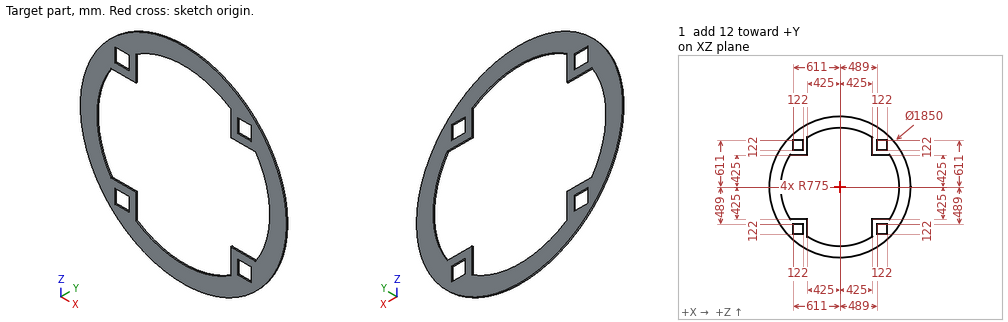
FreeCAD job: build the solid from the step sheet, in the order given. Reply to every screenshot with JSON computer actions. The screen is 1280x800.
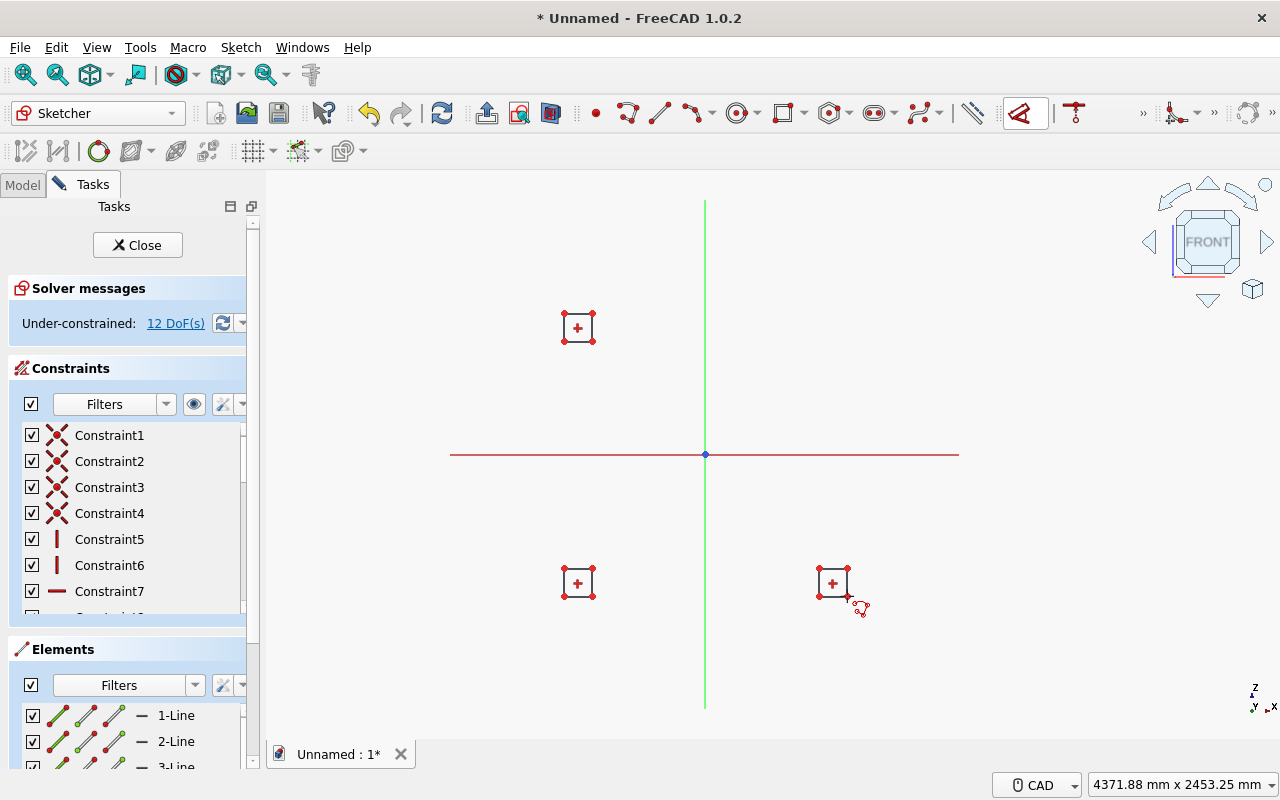
{"action": "left_click", "coordinate": [555, 553]}
{"action": "left_click", "coordinate": [607, 553]}
{"action": "left_click", "coordinate": [607, 605]}
{"action": "right_click", "coordinate": [607, 605]}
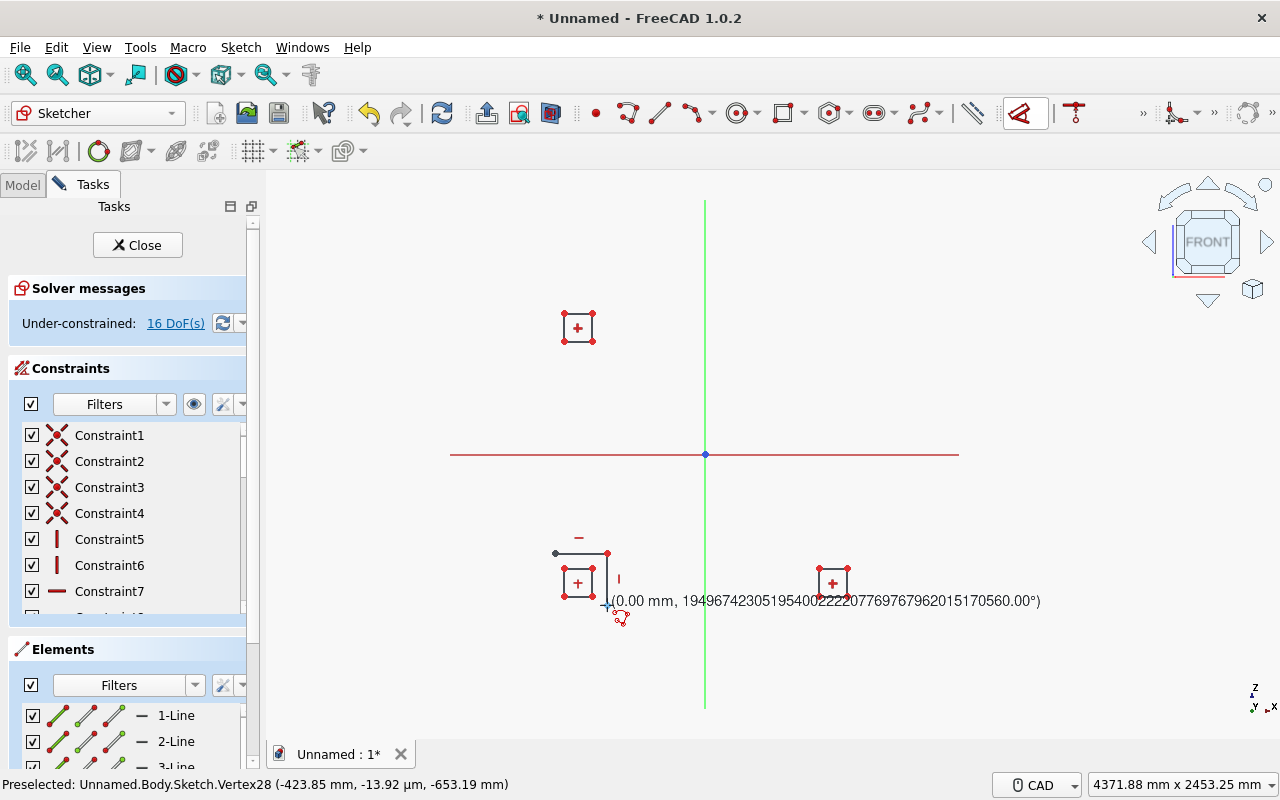
{"action": "left_click", "coordinate": [804, 605]}
{"action": "left_click", "coordinate": [804, 553]}
{"action": "left_click", "coordinate": [856, 553]}
{"action": "right_click", "coordinate": [856, 553]}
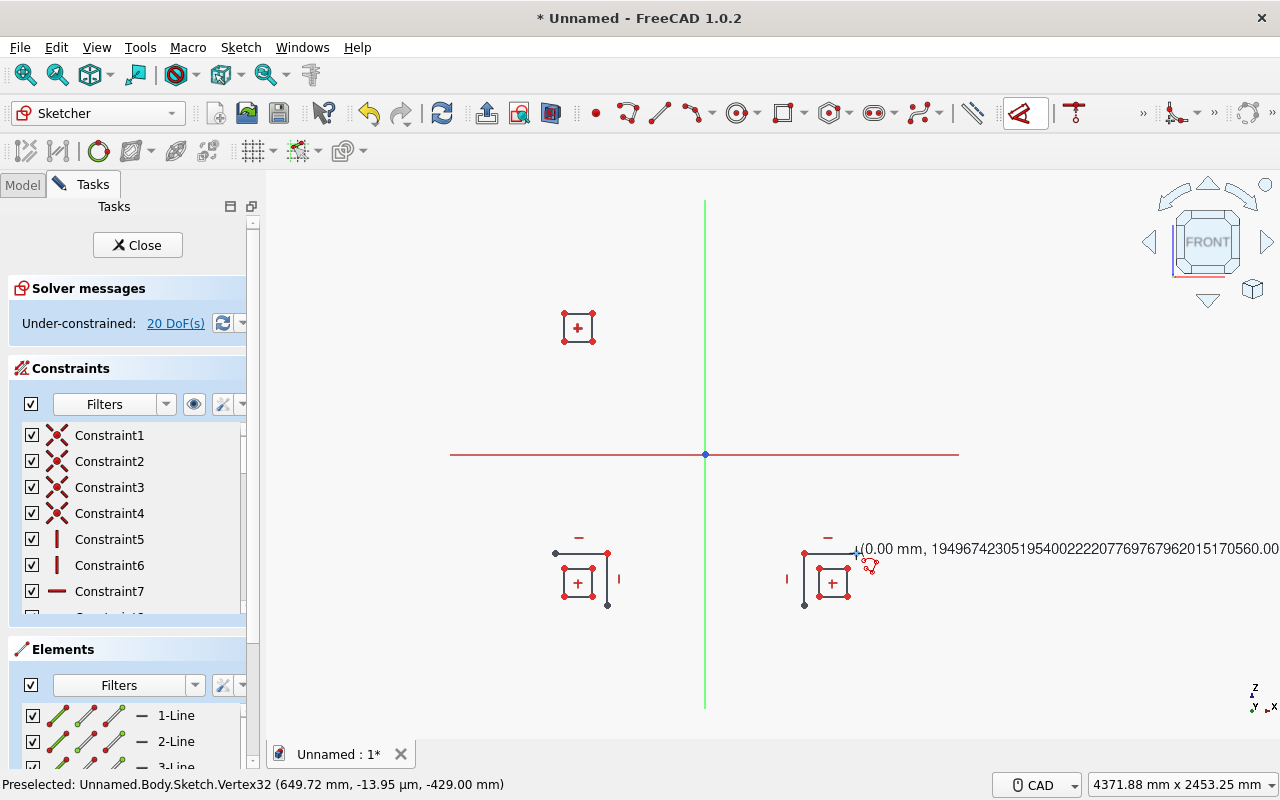
{"action": "left_click", "coordinate": [856, 356]}
{"action": "left_click", "coordinate": [804, 356]}
{"action": "left_click", "coordinate": [804, 304]}
{"action": "right_click", "coordinate": [804, 304]}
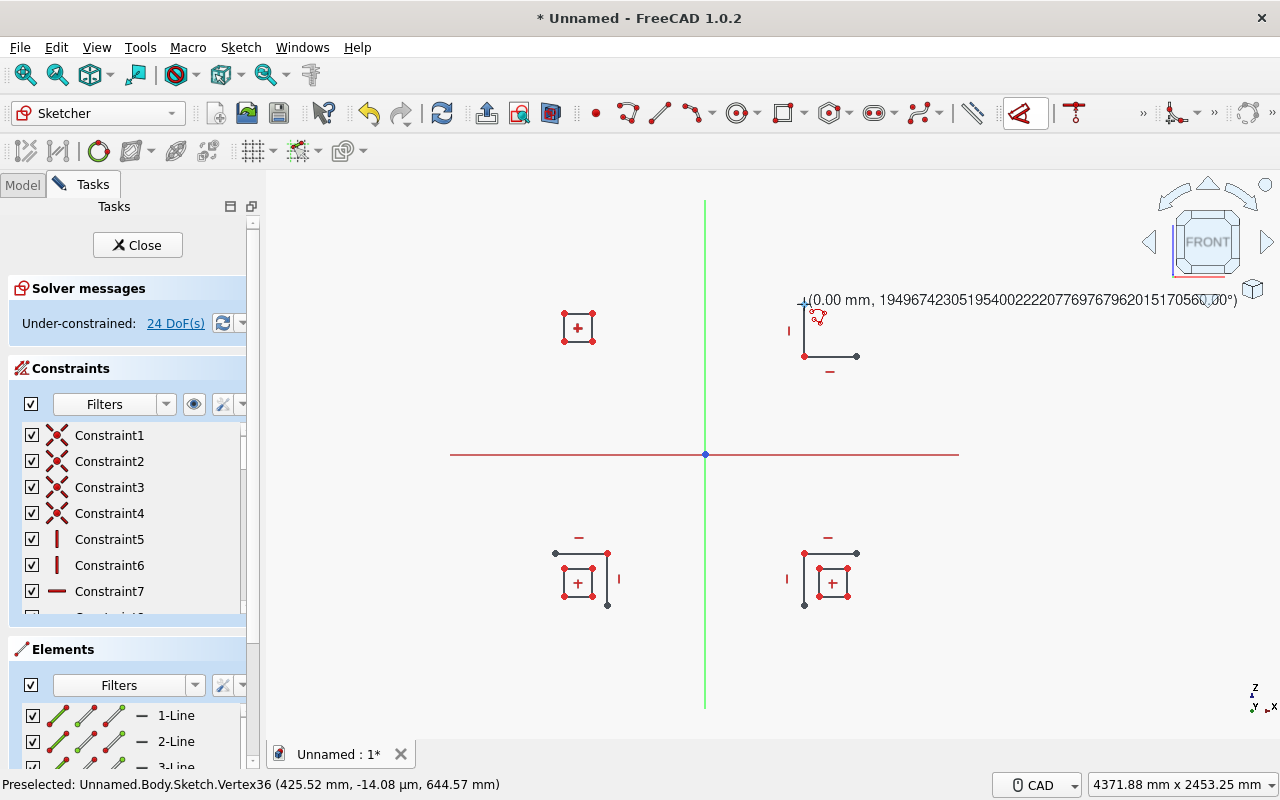
{"action": "left_click", "coordinate": [607, 304]}
{"action": "left_click", "coordinate": [607, 356]}
{"action": "left_click", "coordinate": [555, 356]}
{"action": "right_click", "coordinate": [555, 356]}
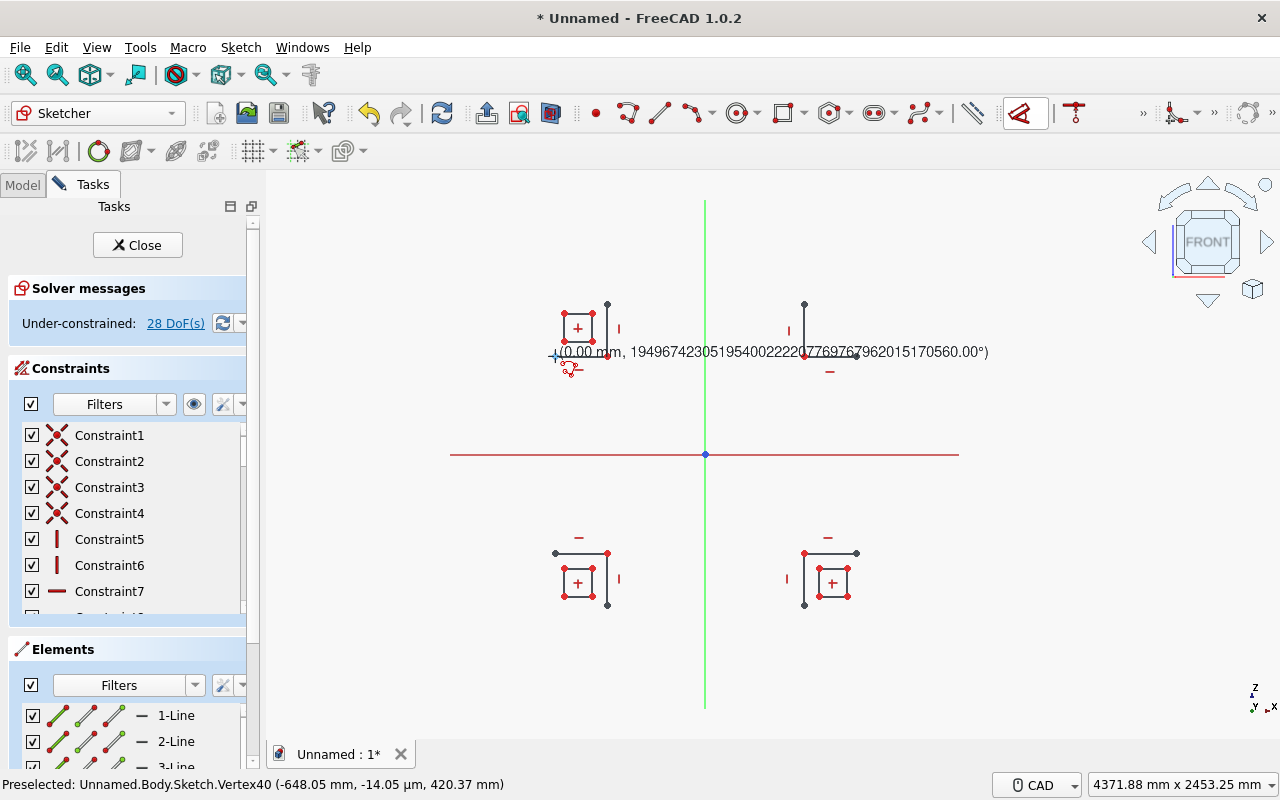
{"action": "left_click", "coordinate": [692, 114]}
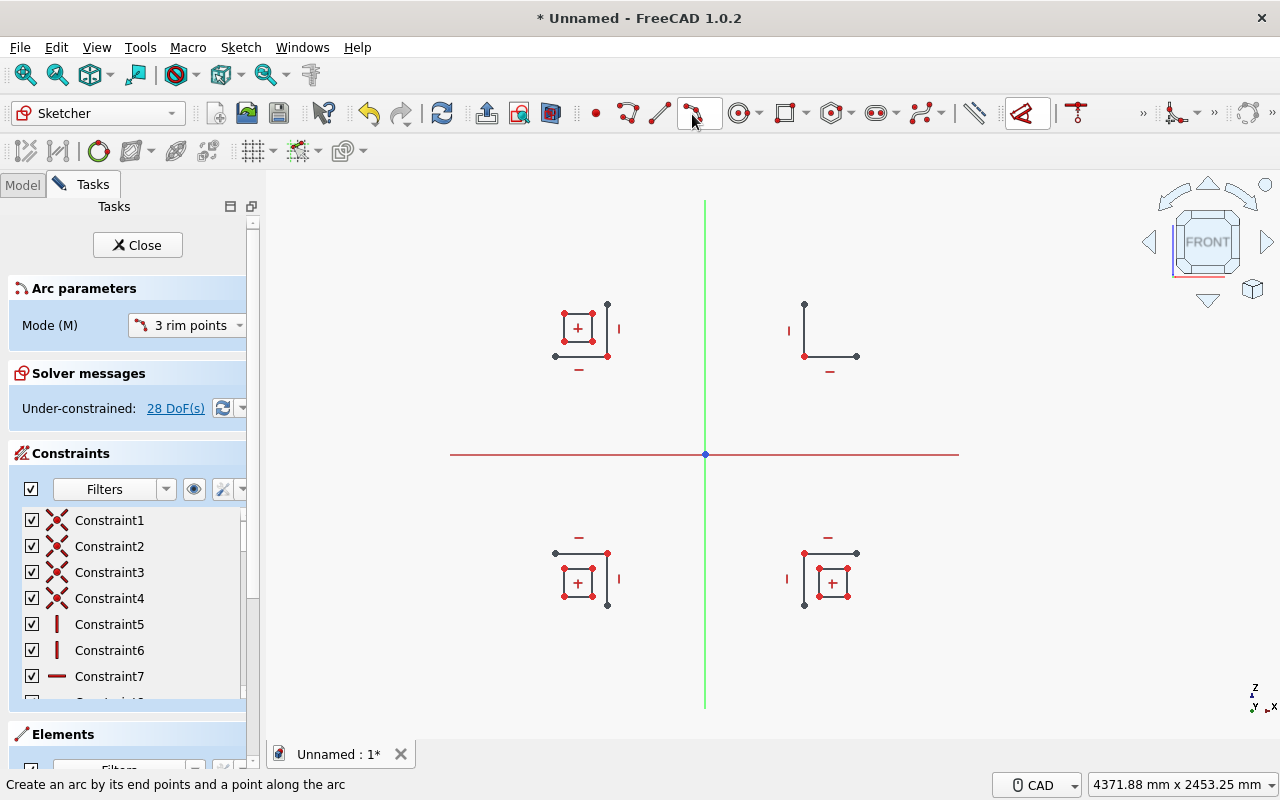
{"action": "left_click", "coordinate": [607, 606]}
{"action": "left_click", "coordinate": [804, 606]}
{"action": "left_click", "coordinate": [684, 633]}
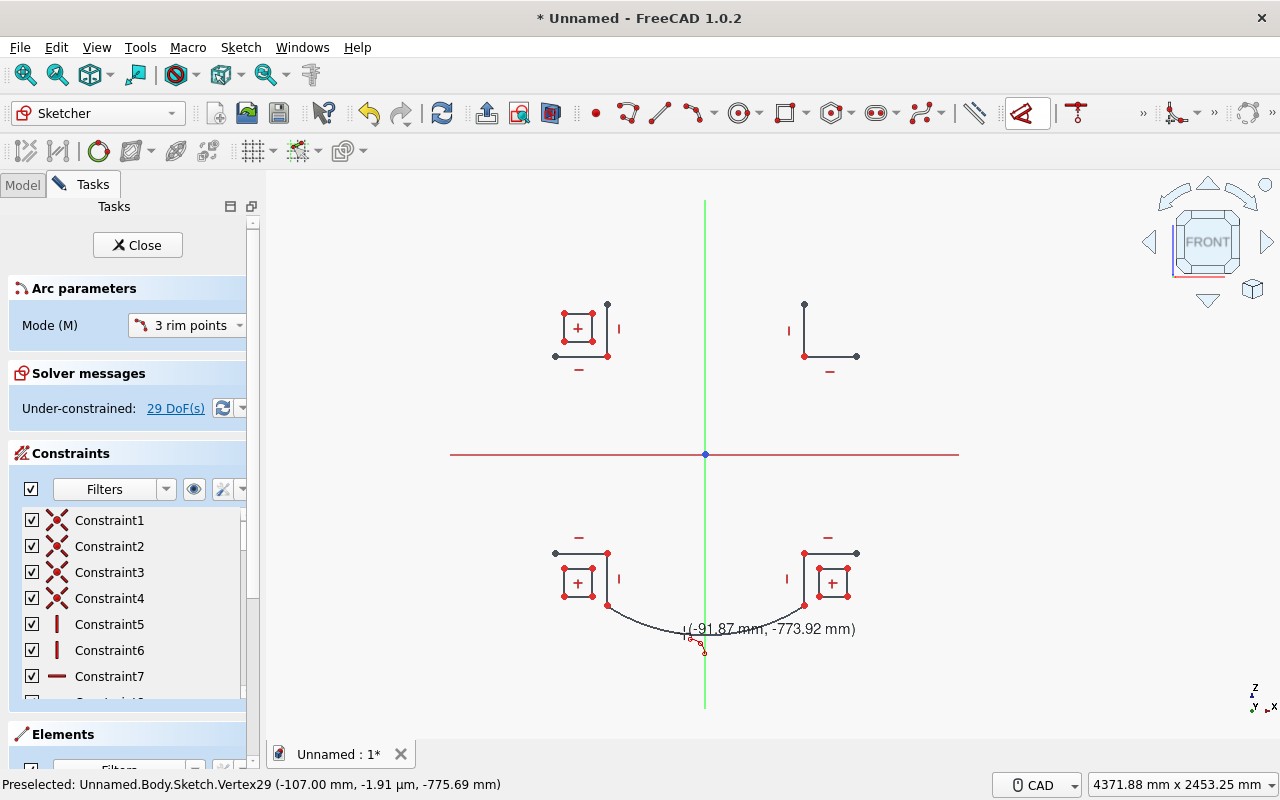
{"action": "left_click", "coordinate": [856, 554]}
{"action": "left_click", "coordinate": [856, 357]}
{"action": "left_click", "coordinate": [884, 475]}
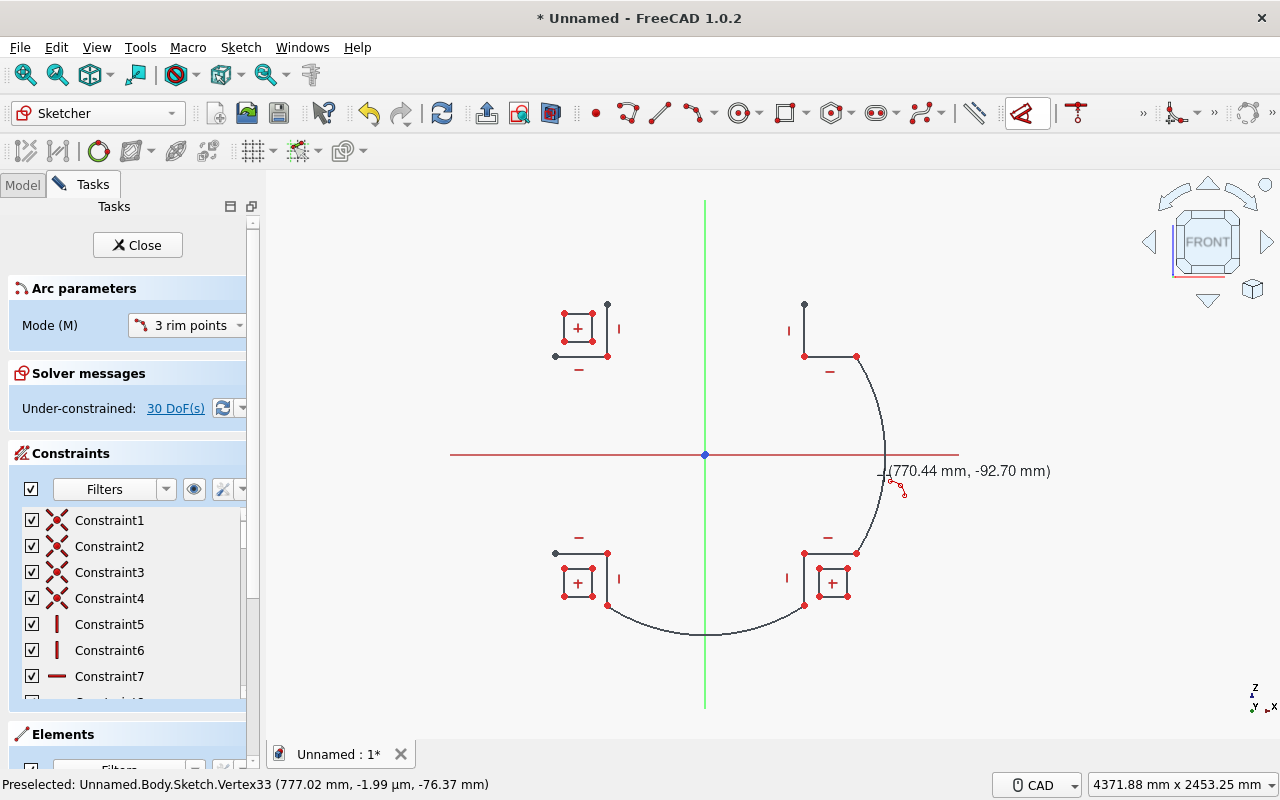
{"action": "left_click", "coordinate": [804, 305]}
{"action": "left_click", "coordinate": [607, 305]}
{"action": "left_click", "coordinate": [726, 276]}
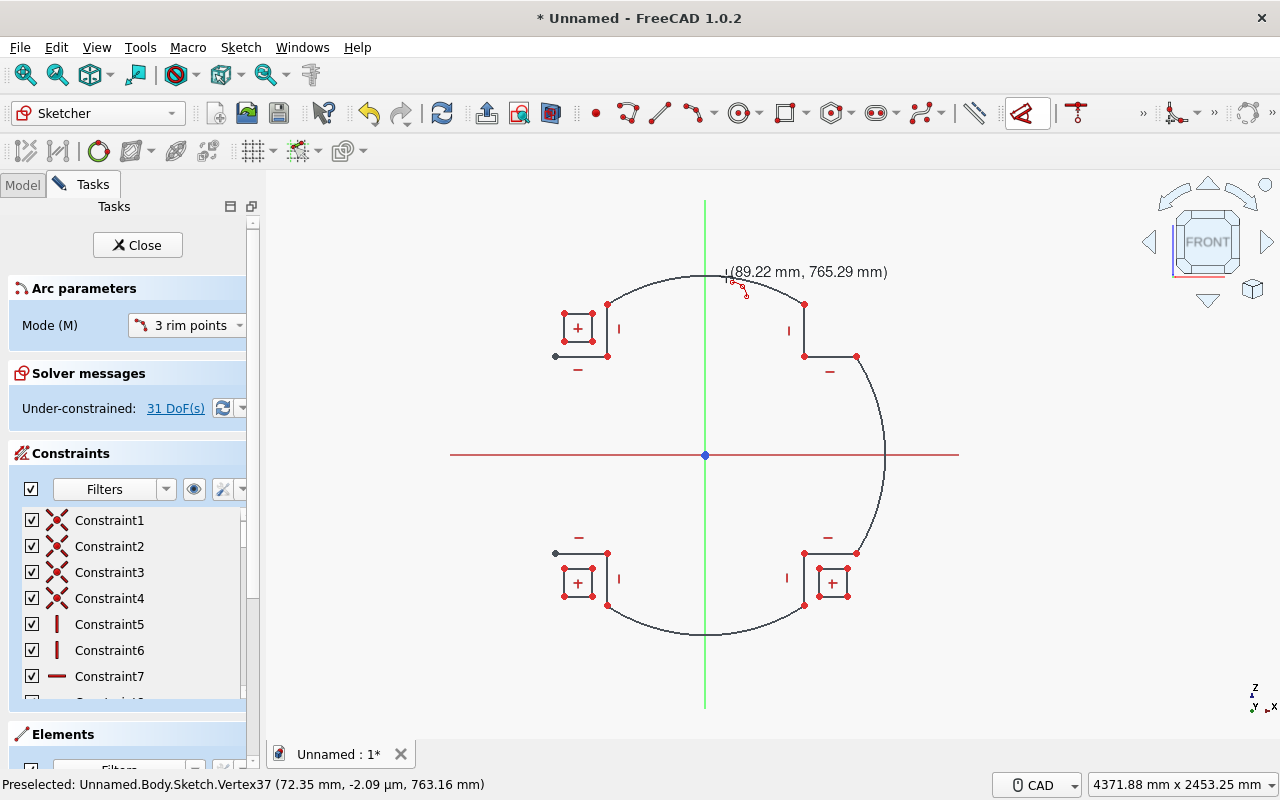
{"action": "left_click", "coordinate": [555, 357]}
{"action": "left_click", "coordinate": [555, 554]}
{"action": "left_click", "coordinate": [527, 434]}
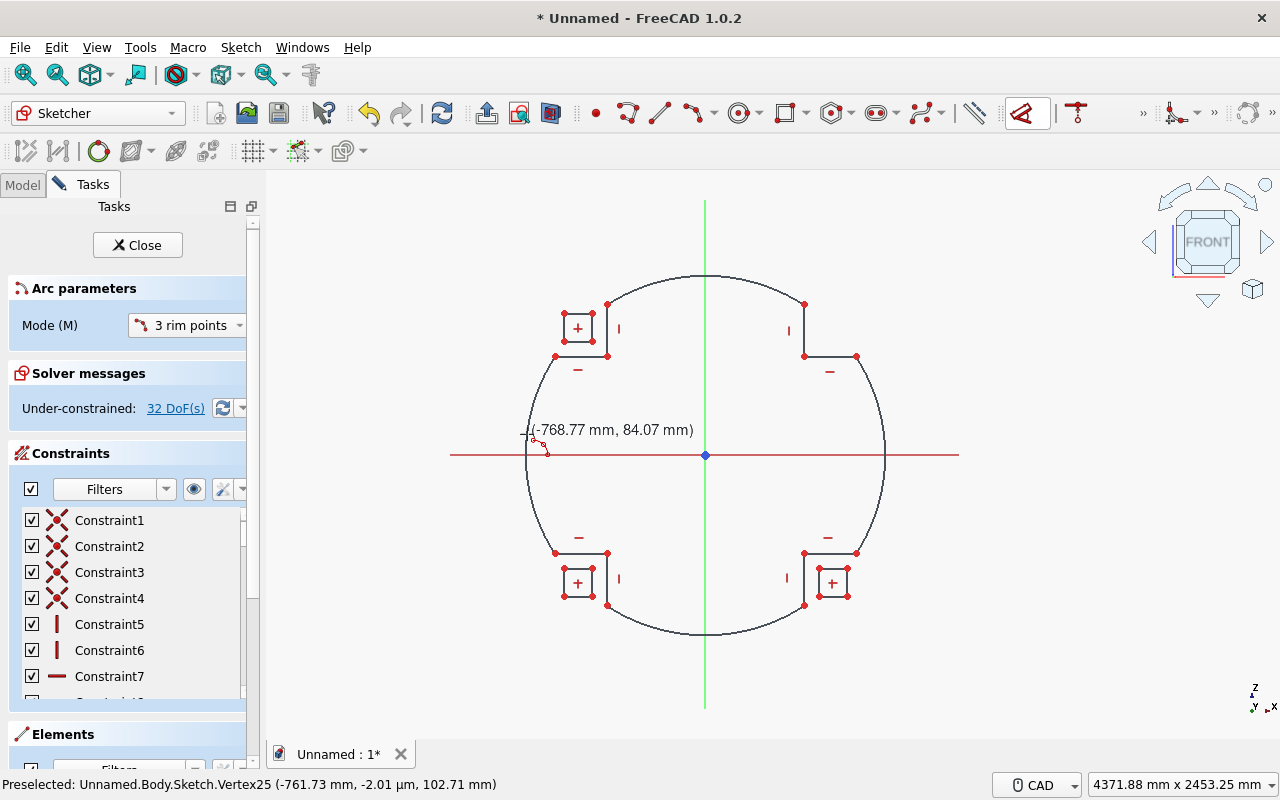
{"action": "key", "text": "g r"}